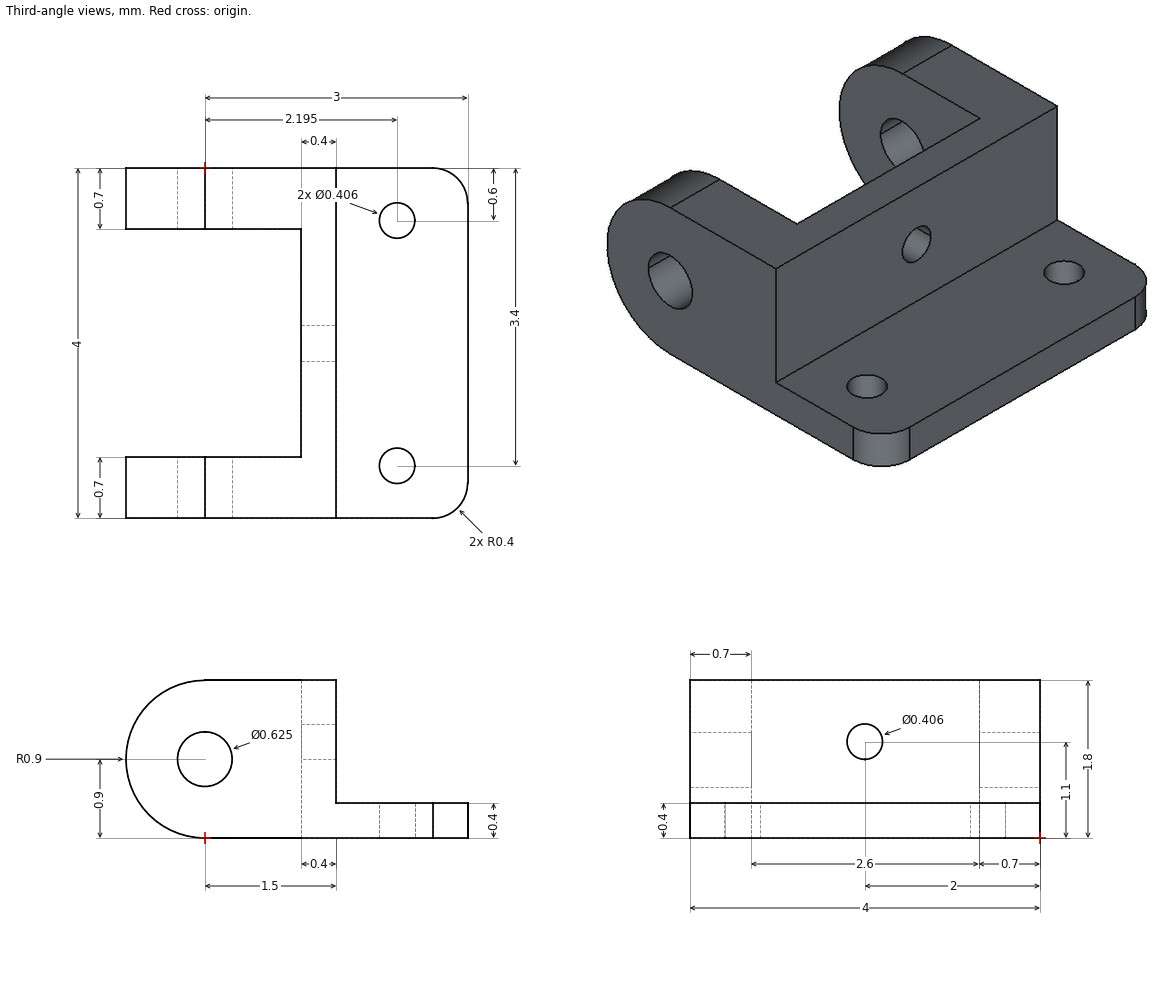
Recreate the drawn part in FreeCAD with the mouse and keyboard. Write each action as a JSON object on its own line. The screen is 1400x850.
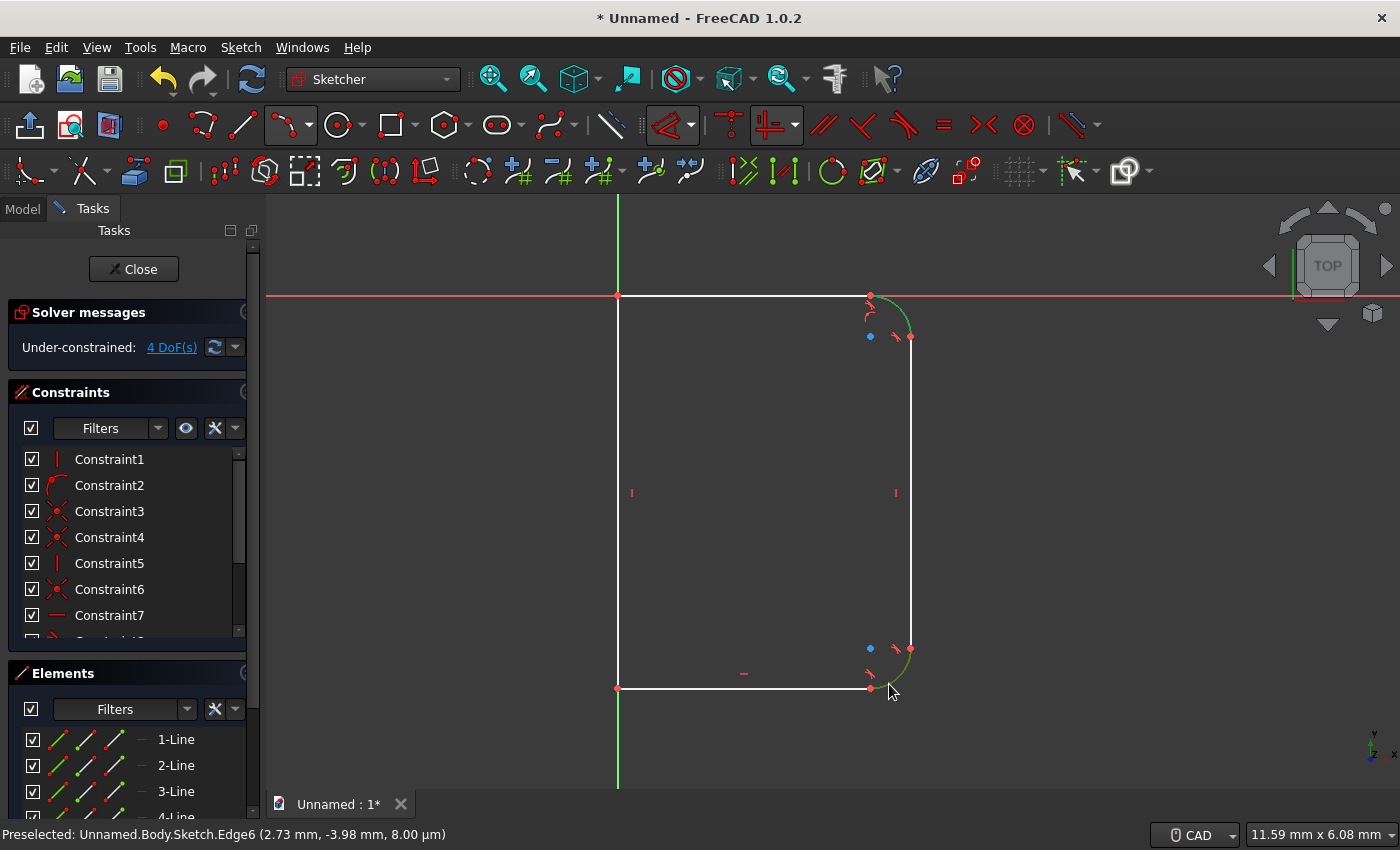
{"action": "key", "text": "e"}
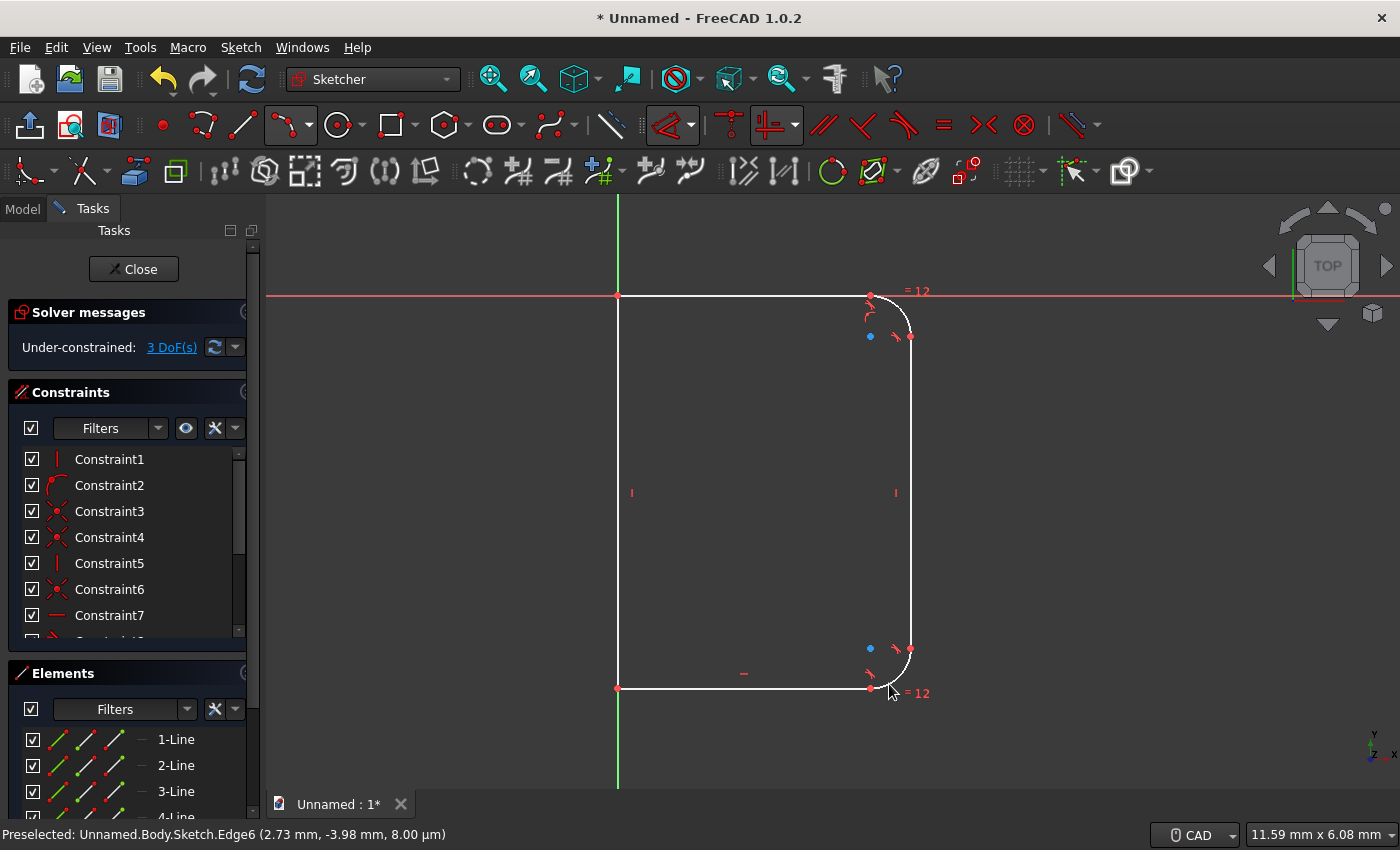
{"action": "key", "text": "d"}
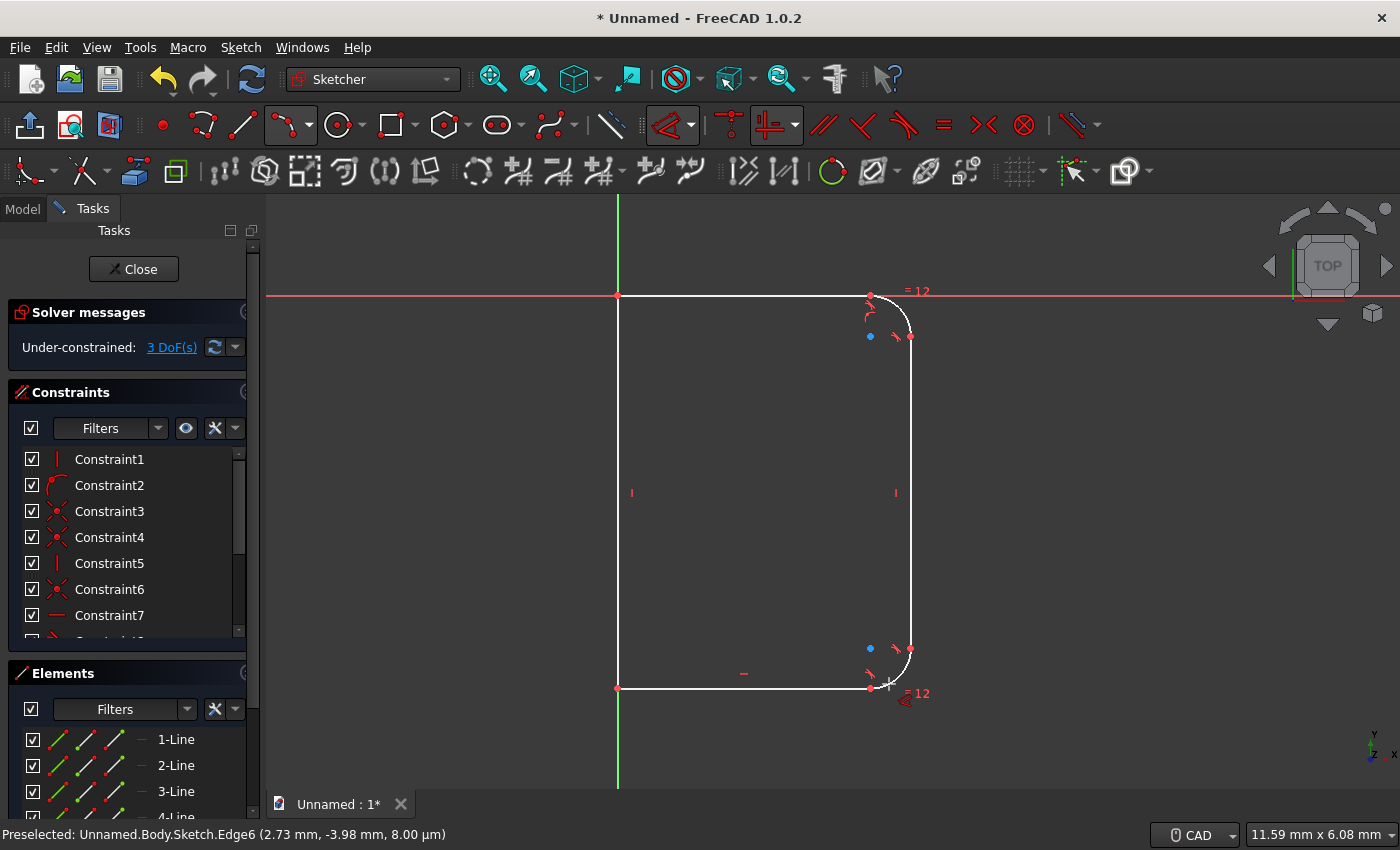
{"action": "left_click", "coordinate": [907, 318]}
{"action": "left_click", "coordinate": [943, 339]}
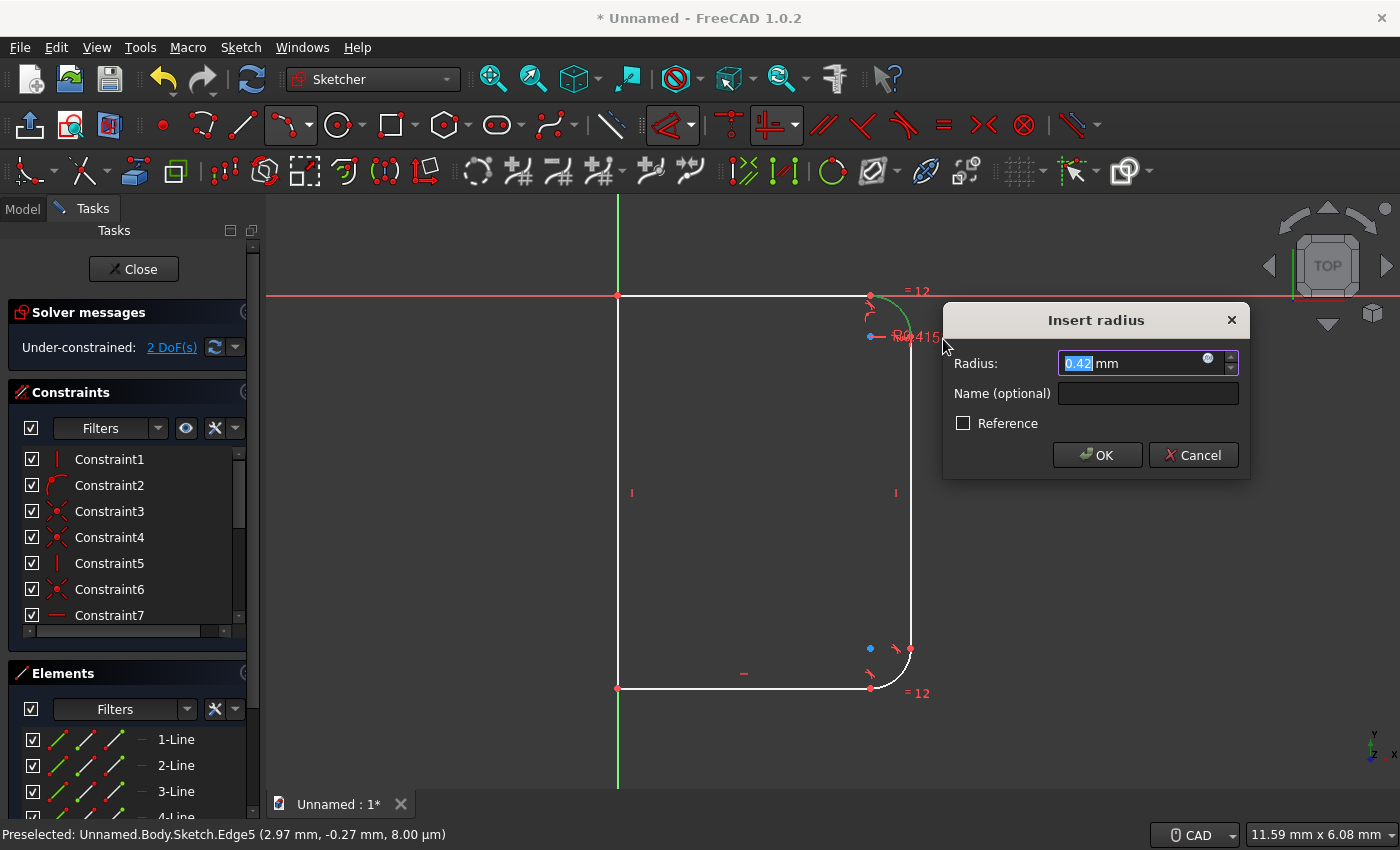
{"action": "type", "text": "0.4"}
{"action": "key", "text": "Return"}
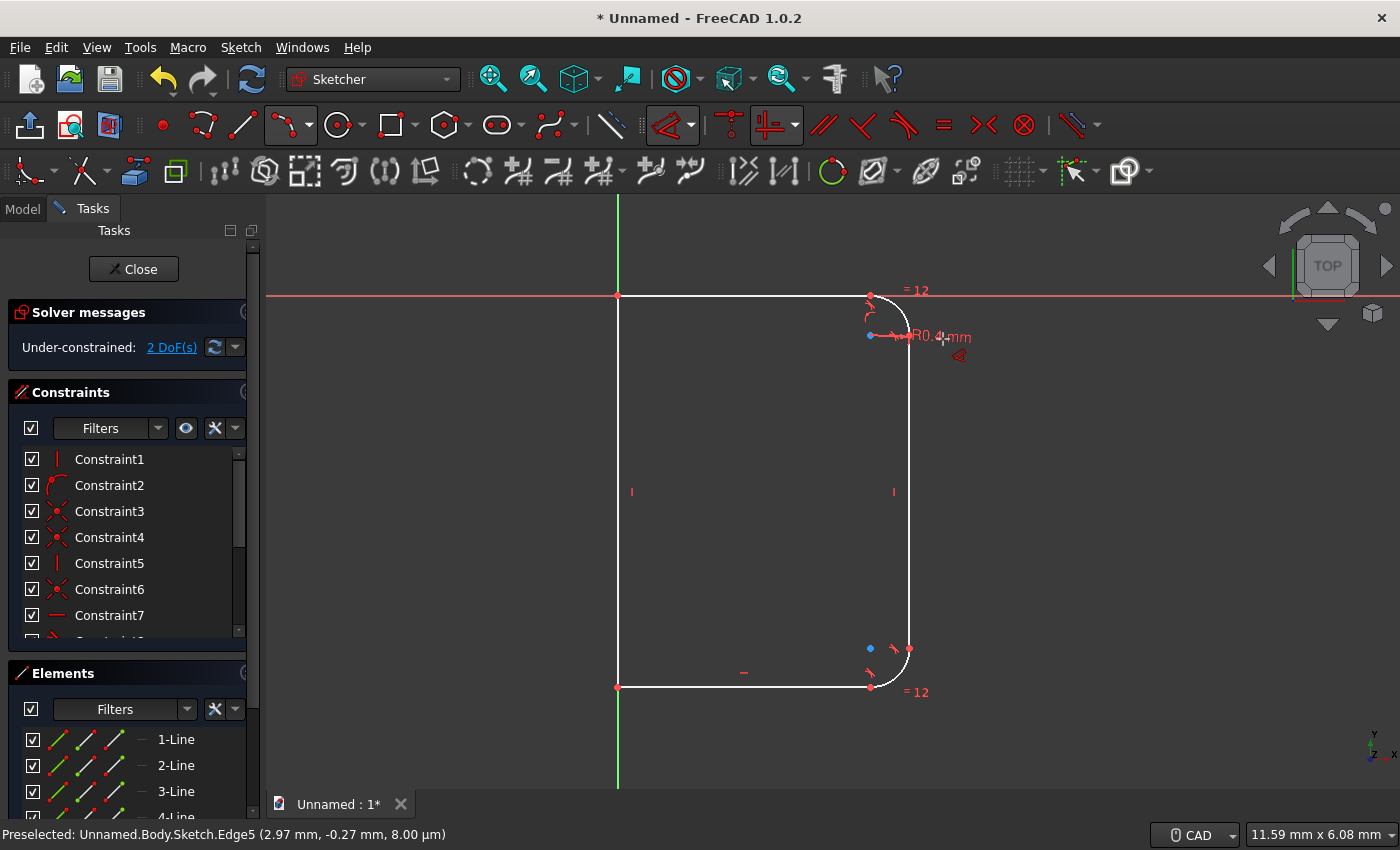
{"action": "left_click", "coordinate": [618, 413]}
{"action": "left_click", "coordinate": [584, 492]}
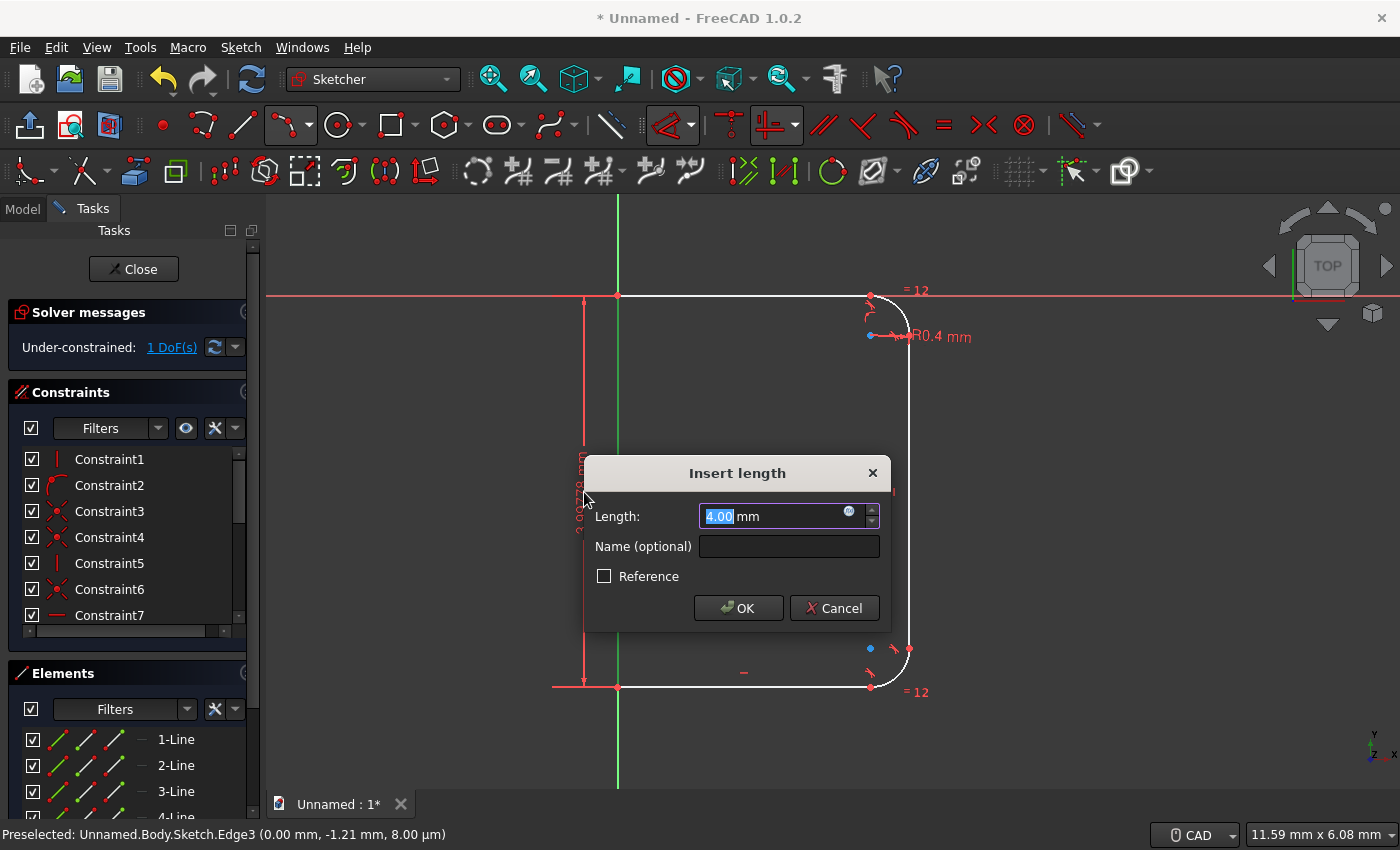
{"action": "type", "text": "4"}
{"action": "key", "text": "Return"}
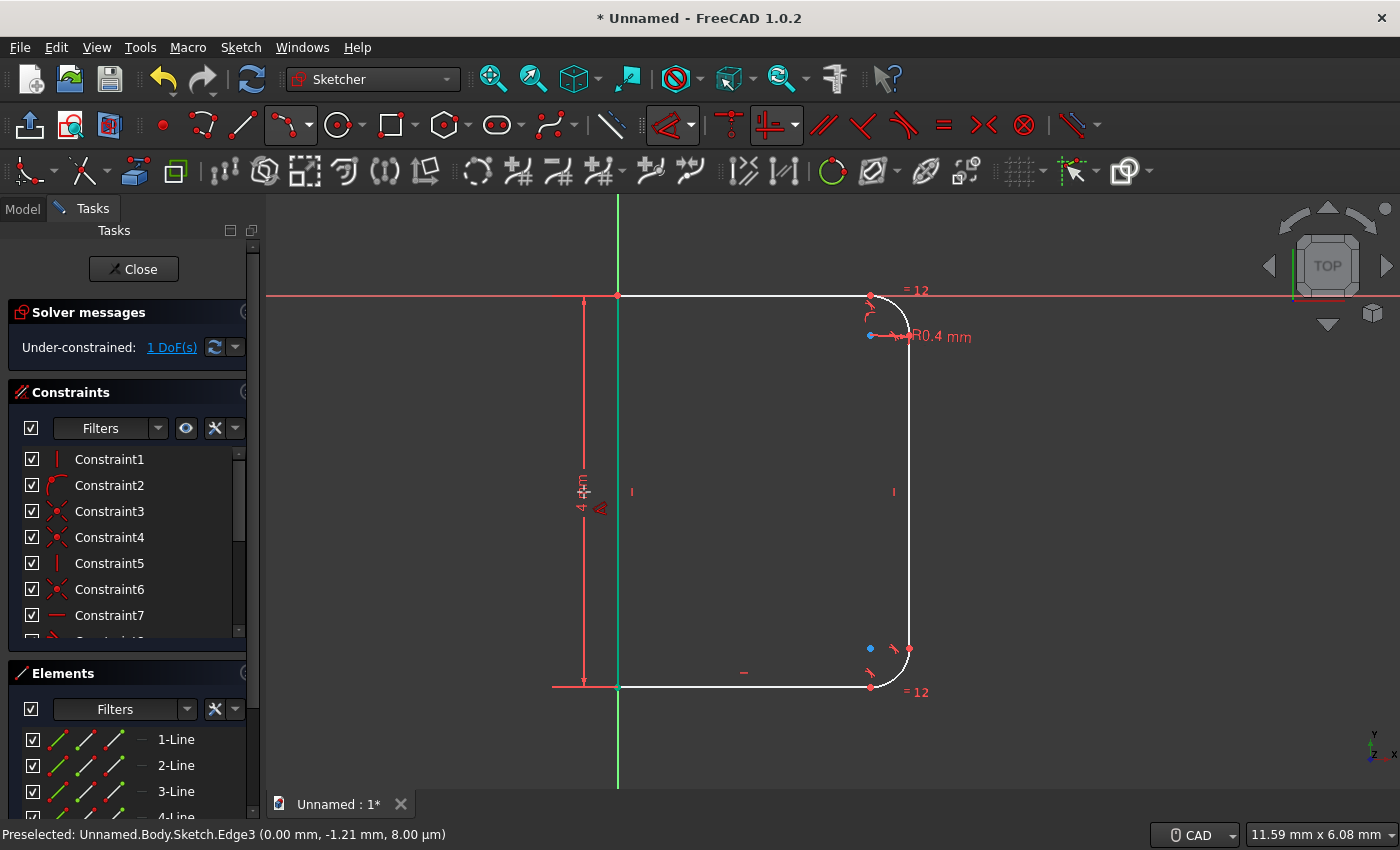
{"action": "left_click", "coordinate": [909, 648]}
{"action": "left_click", "coordinate": [764, 262]}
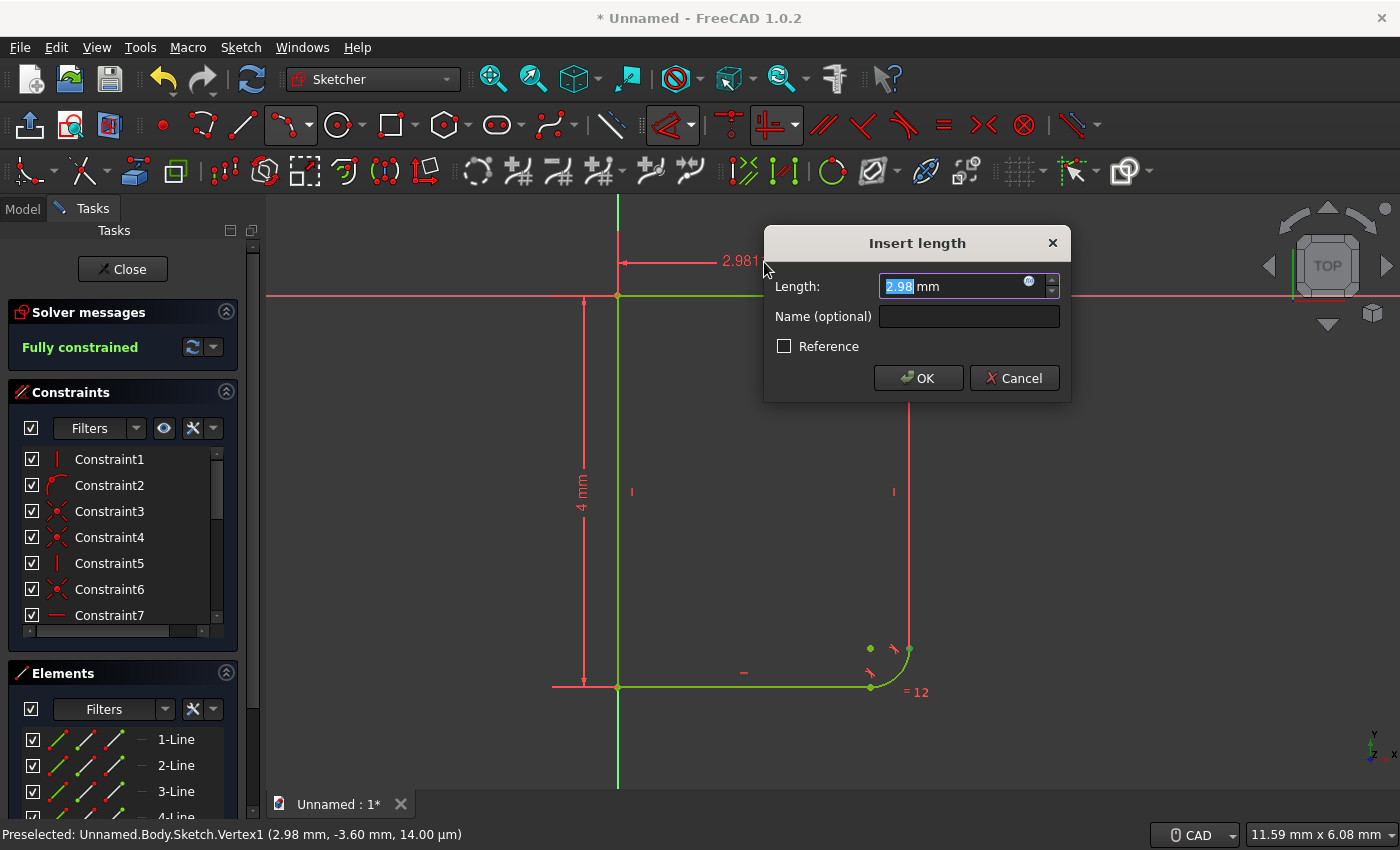
{"action": "type", "text": "3"}
{"action": "key", "text": "Return"}
{"action": "key", "text": "Escape"}